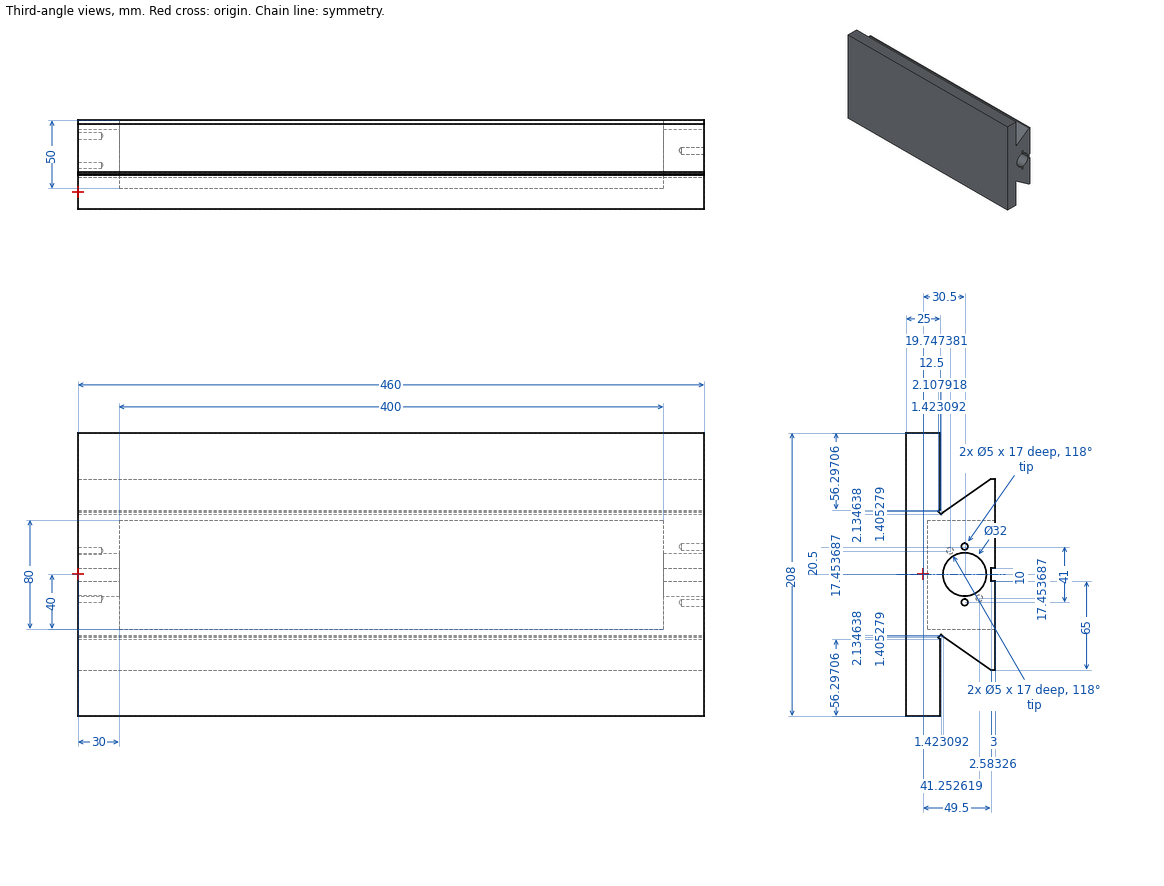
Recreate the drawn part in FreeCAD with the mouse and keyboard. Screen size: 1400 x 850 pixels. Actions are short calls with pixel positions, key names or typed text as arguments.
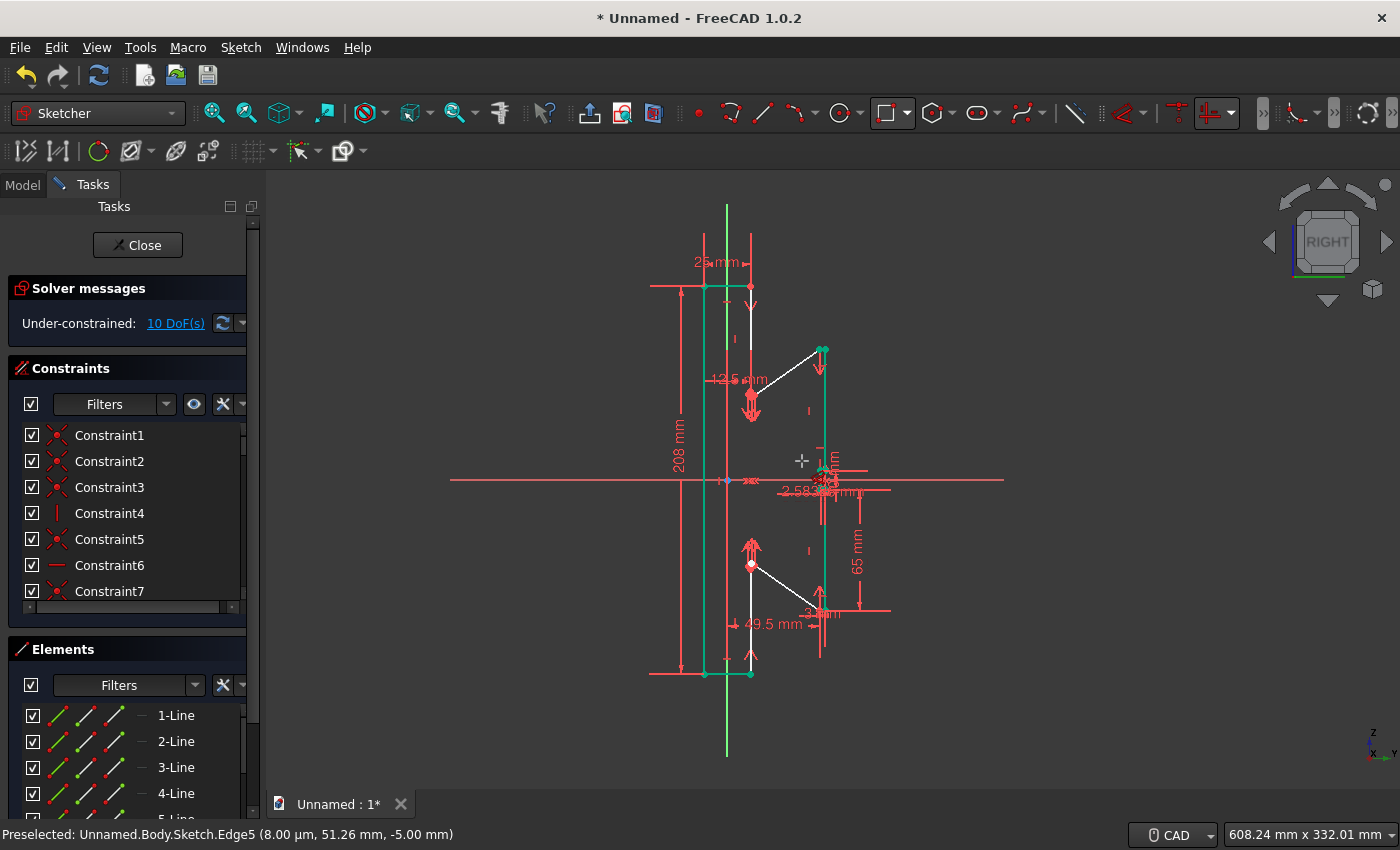
click(751, 360)
click(785, 339)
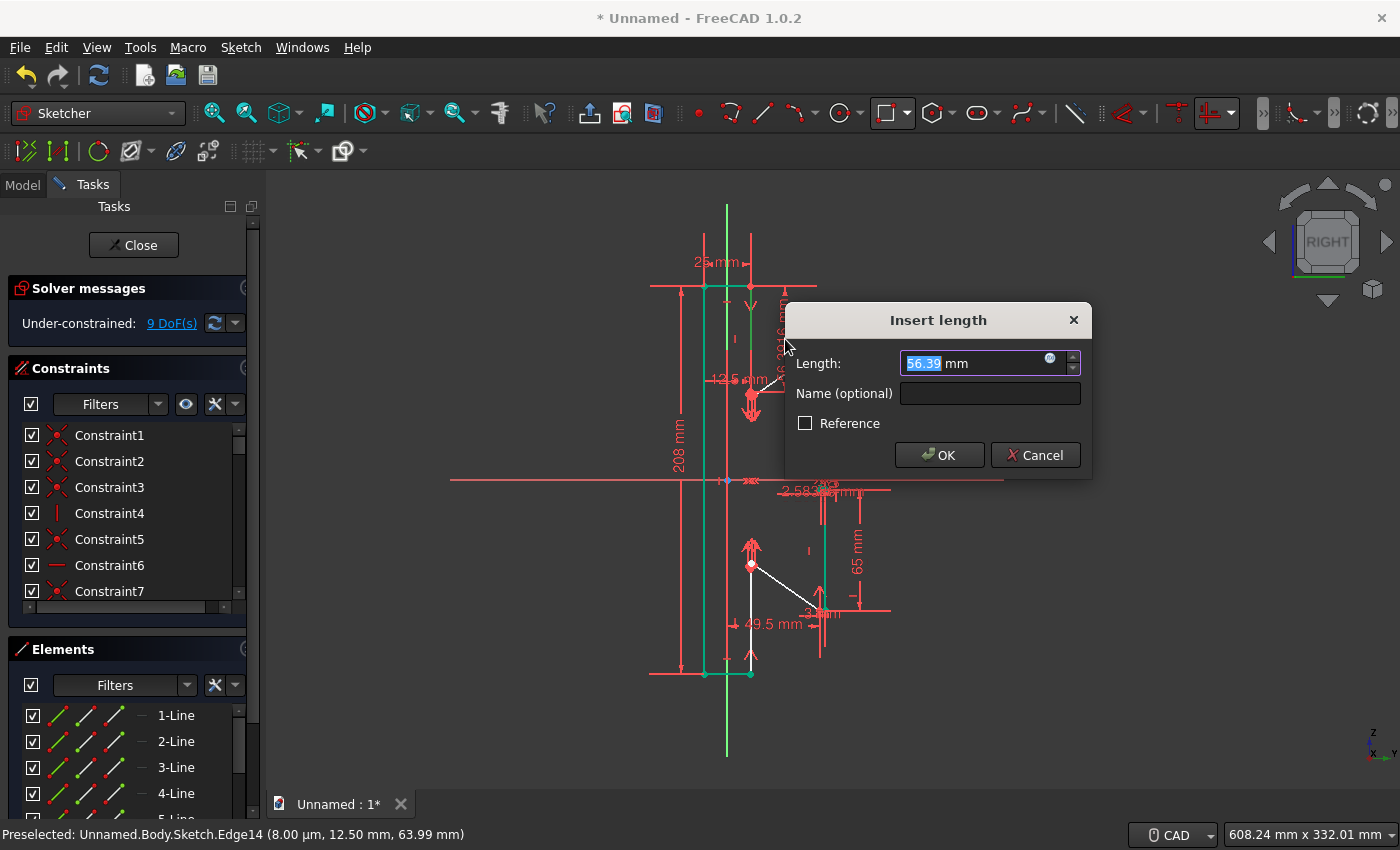
text(56.29706)
key(Return)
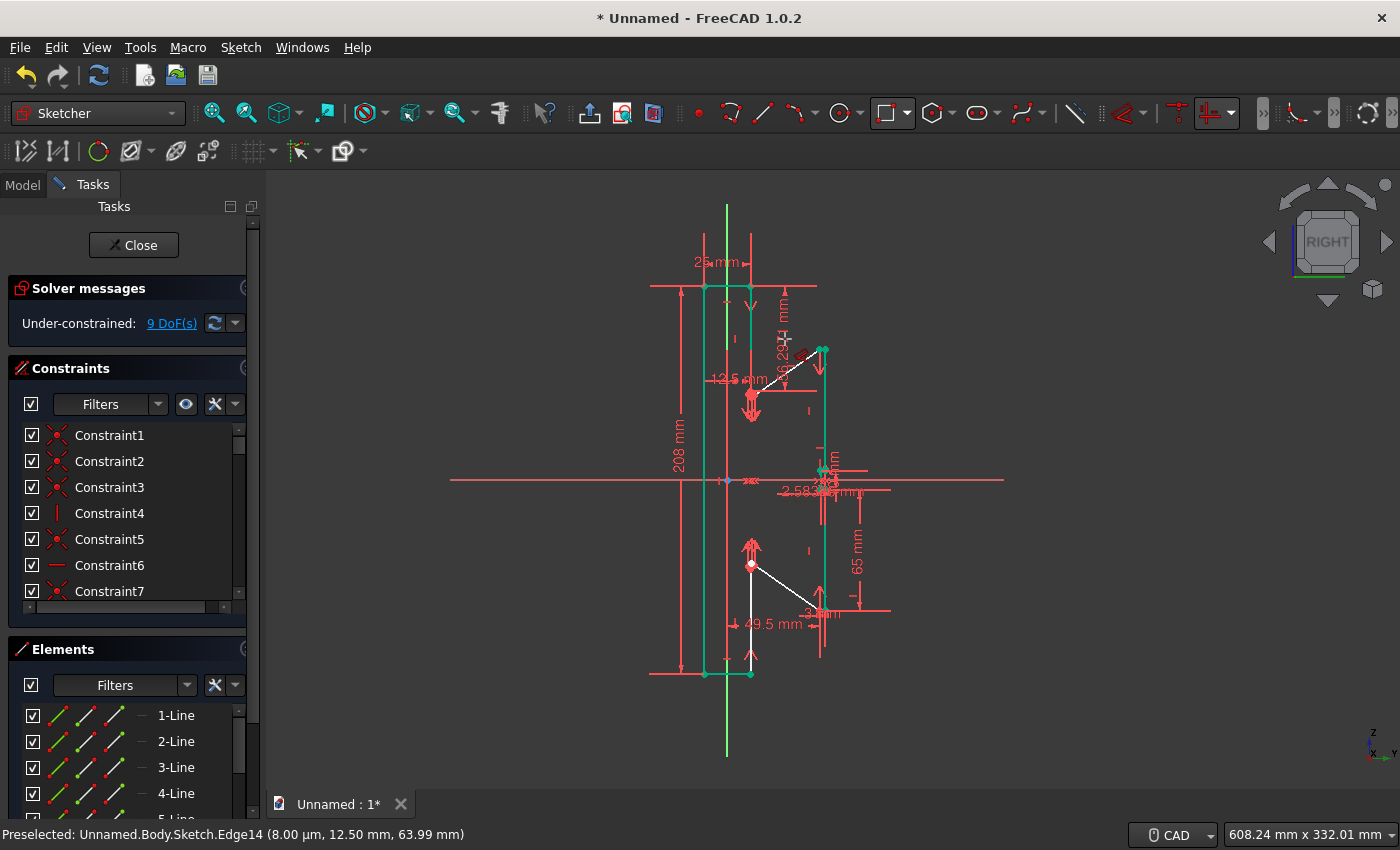
click(751, 643)
click(785, 659)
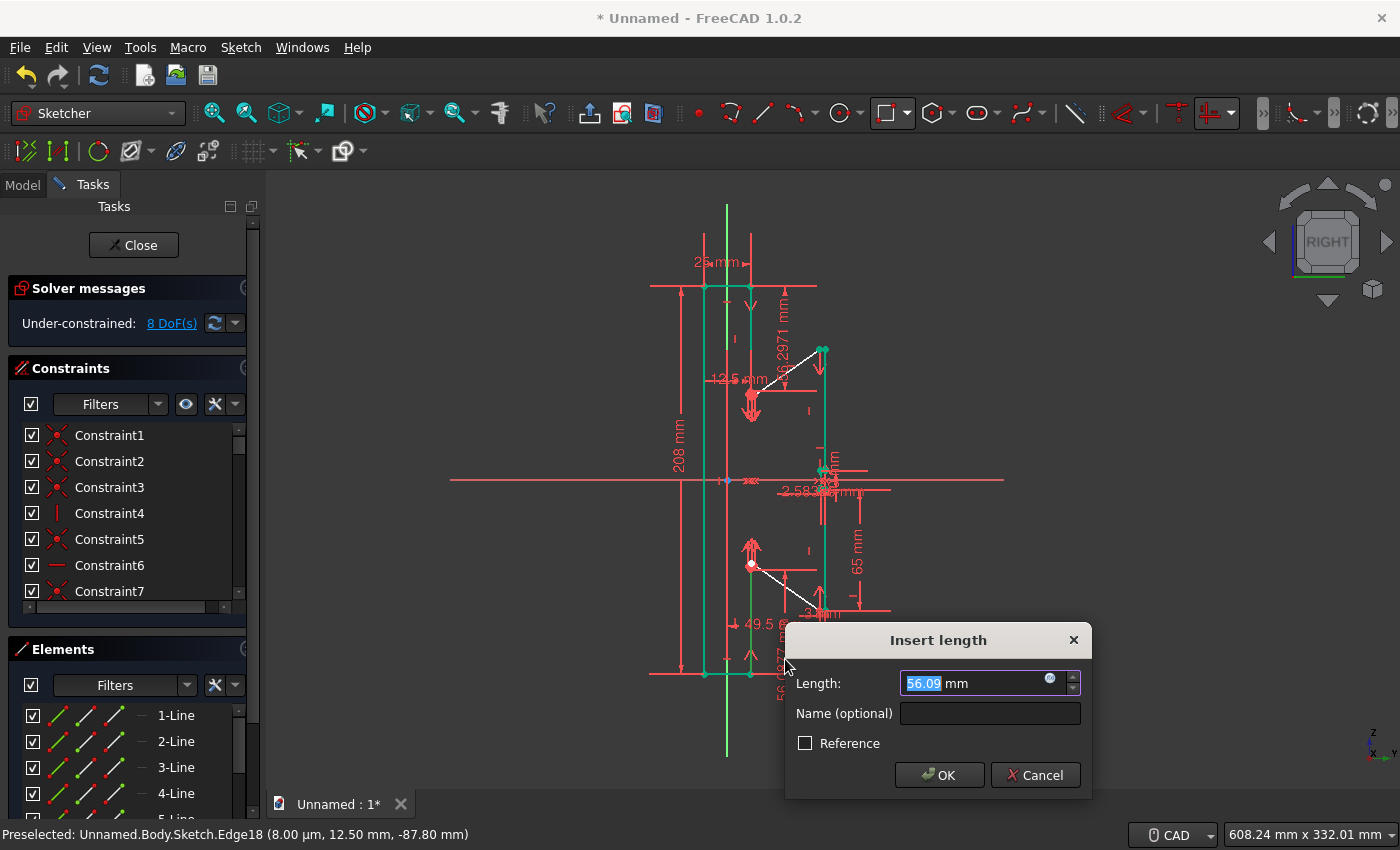
text(56.29706)
key(Return)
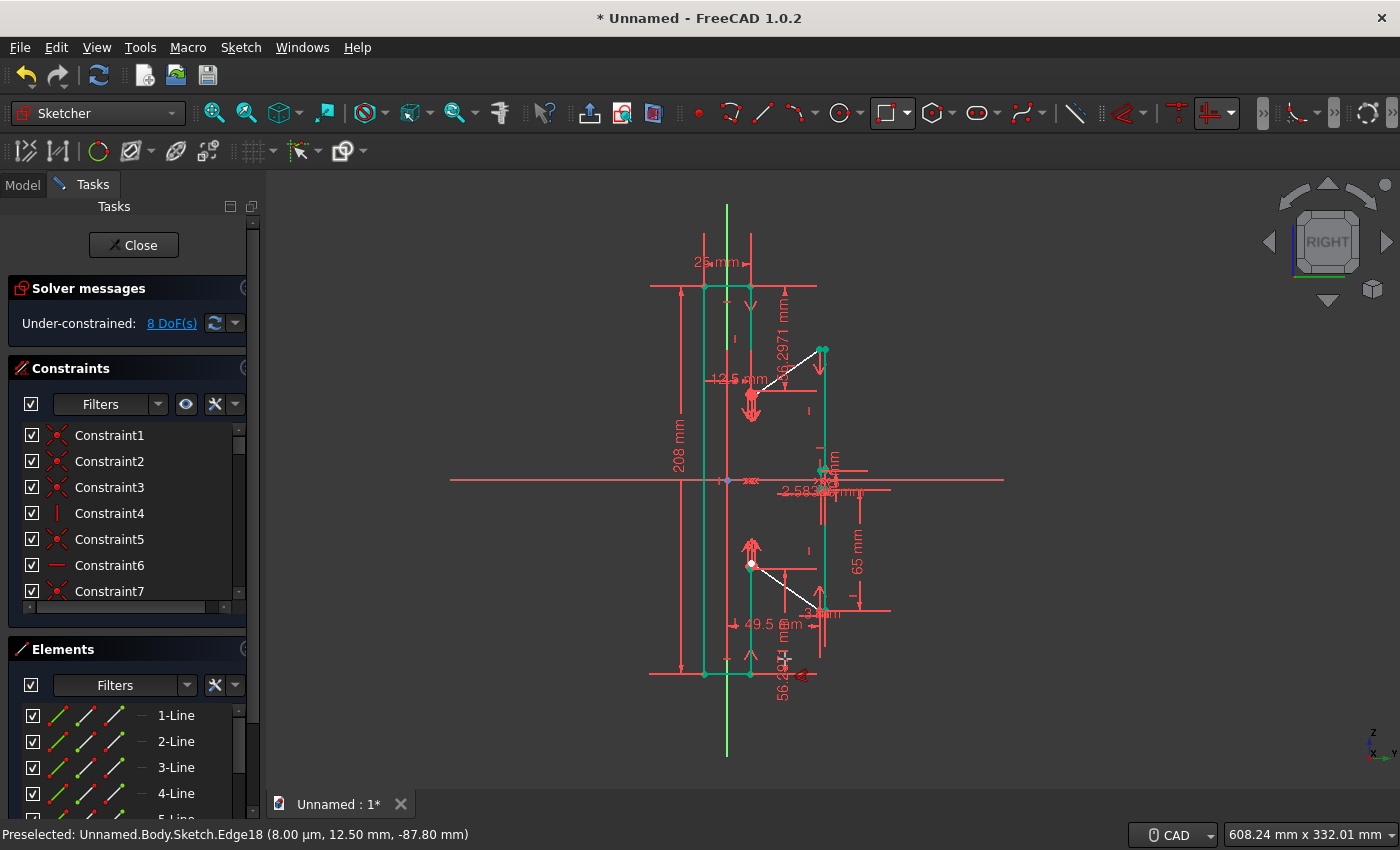
scroll(753, 564, up, 14)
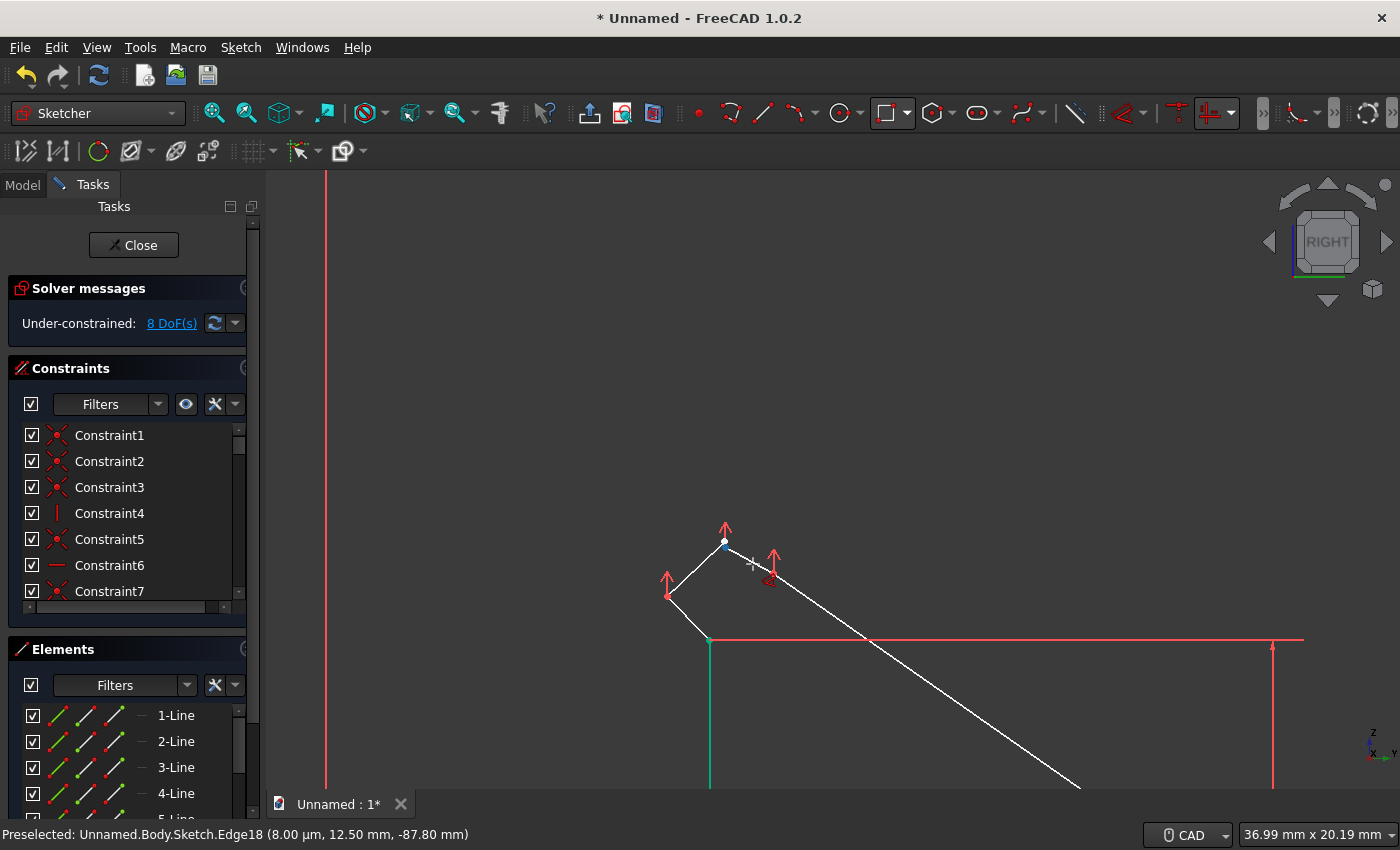
click(750, 561)
click(750, 608)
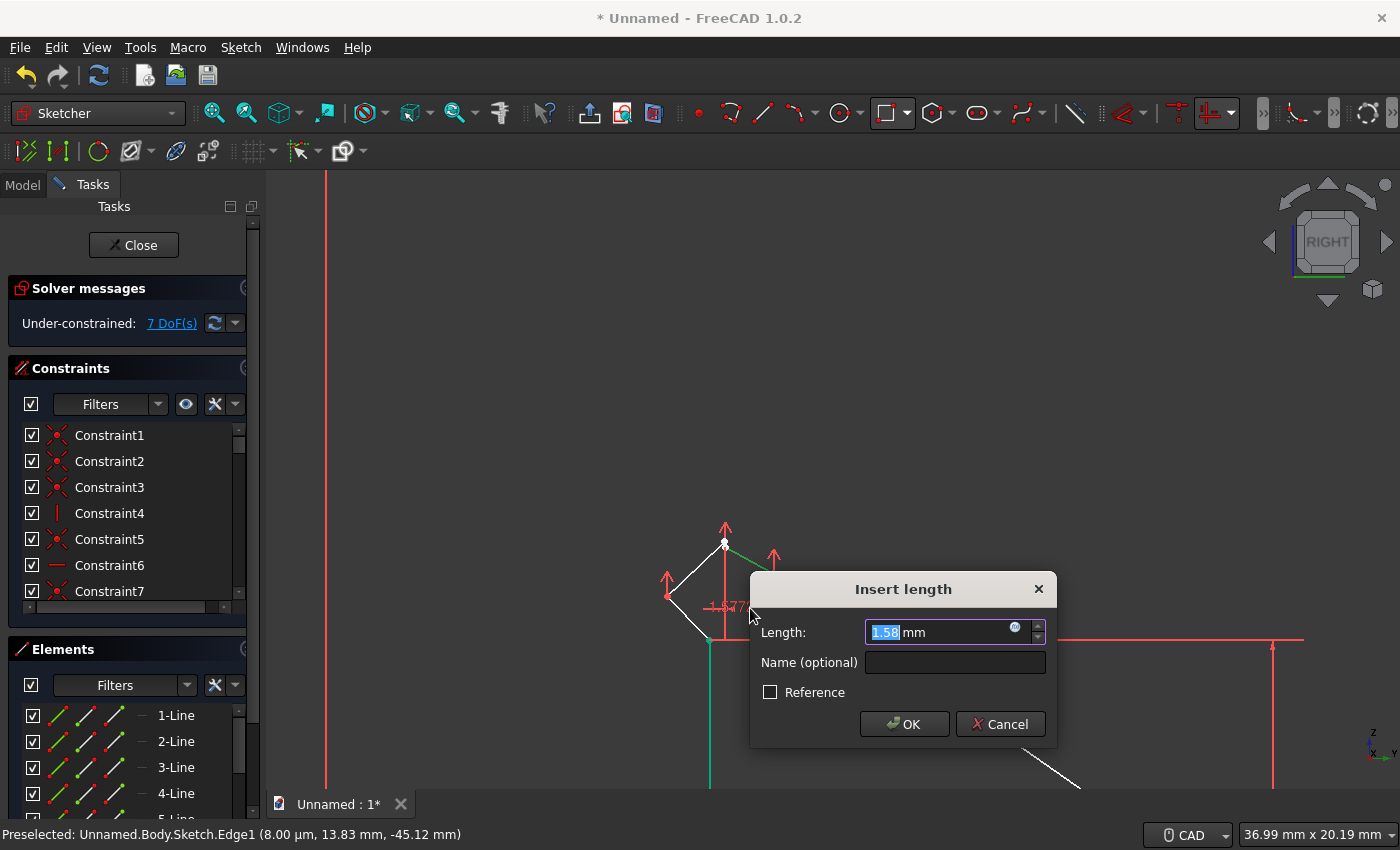
text(1.423092)
key(Return)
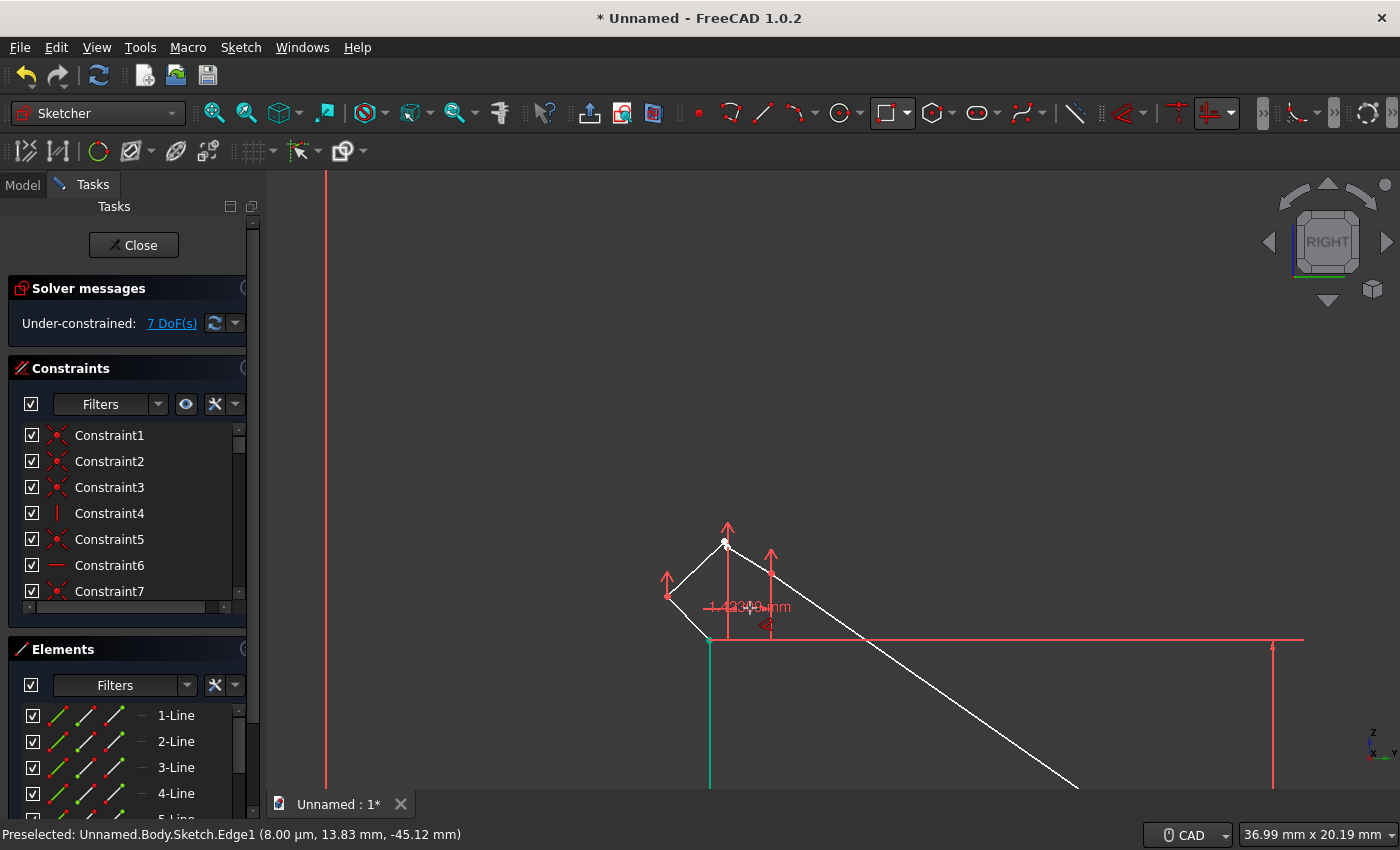
click(741, 555)
click(694, 551)